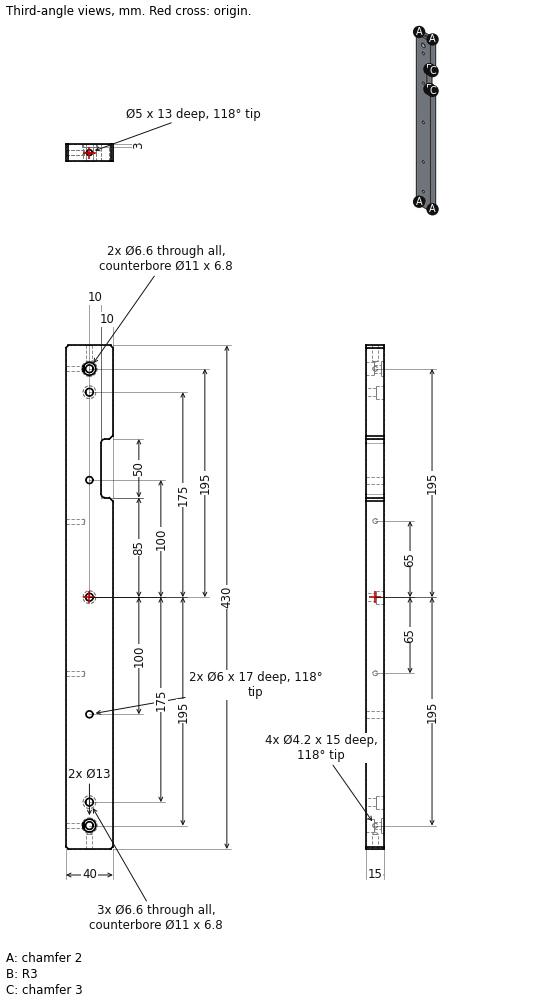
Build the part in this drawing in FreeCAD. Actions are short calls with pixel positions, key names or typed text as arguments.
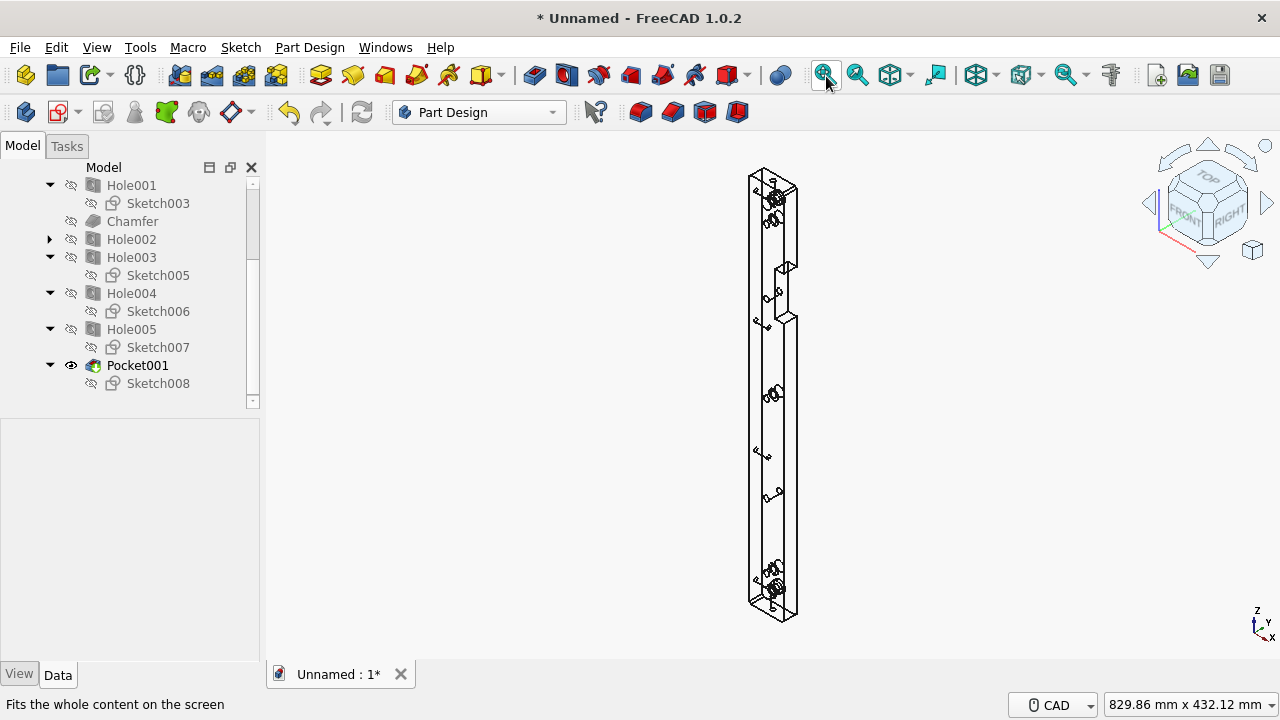
click(782, 314)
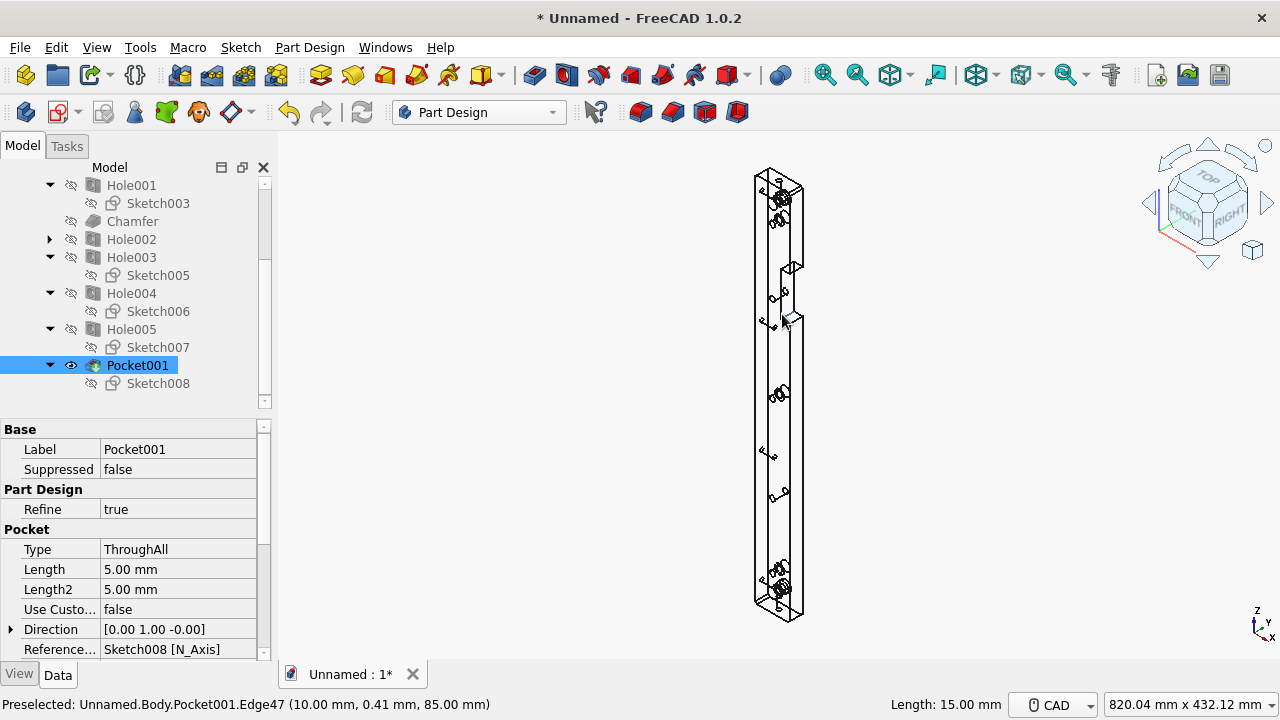
scroll(788, 264, up, 6)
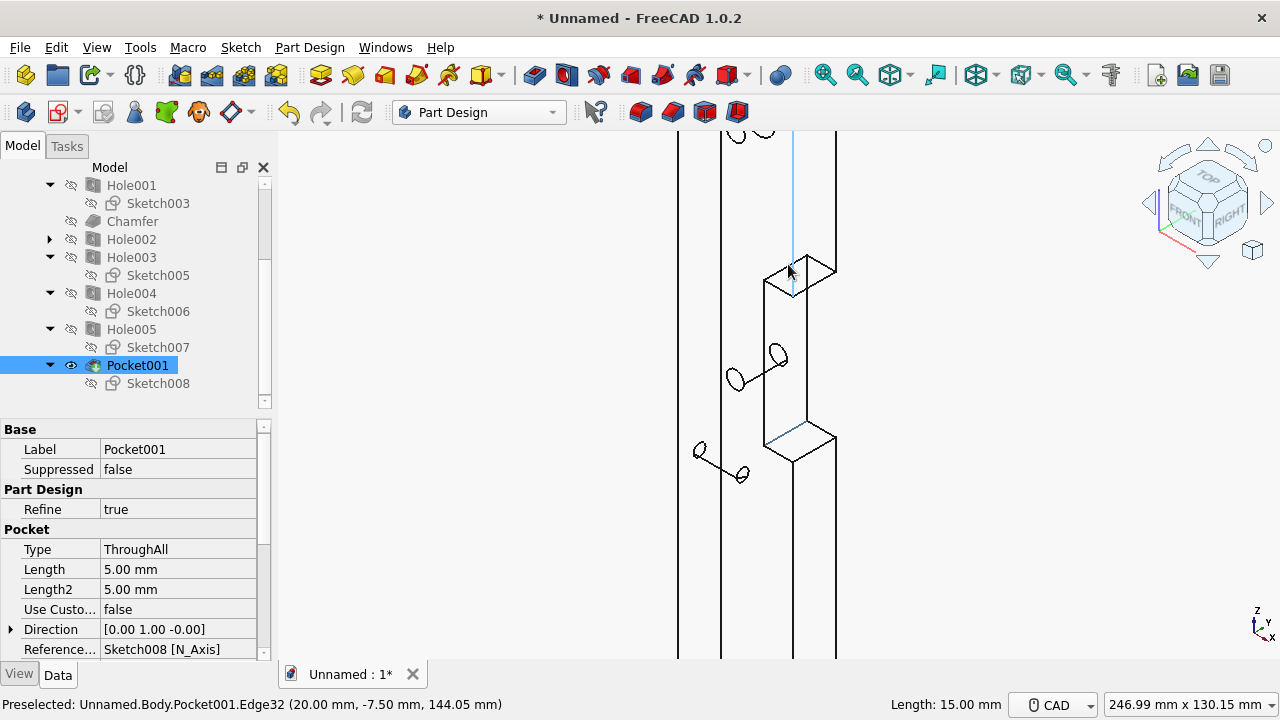
click(786, 267, ctrl)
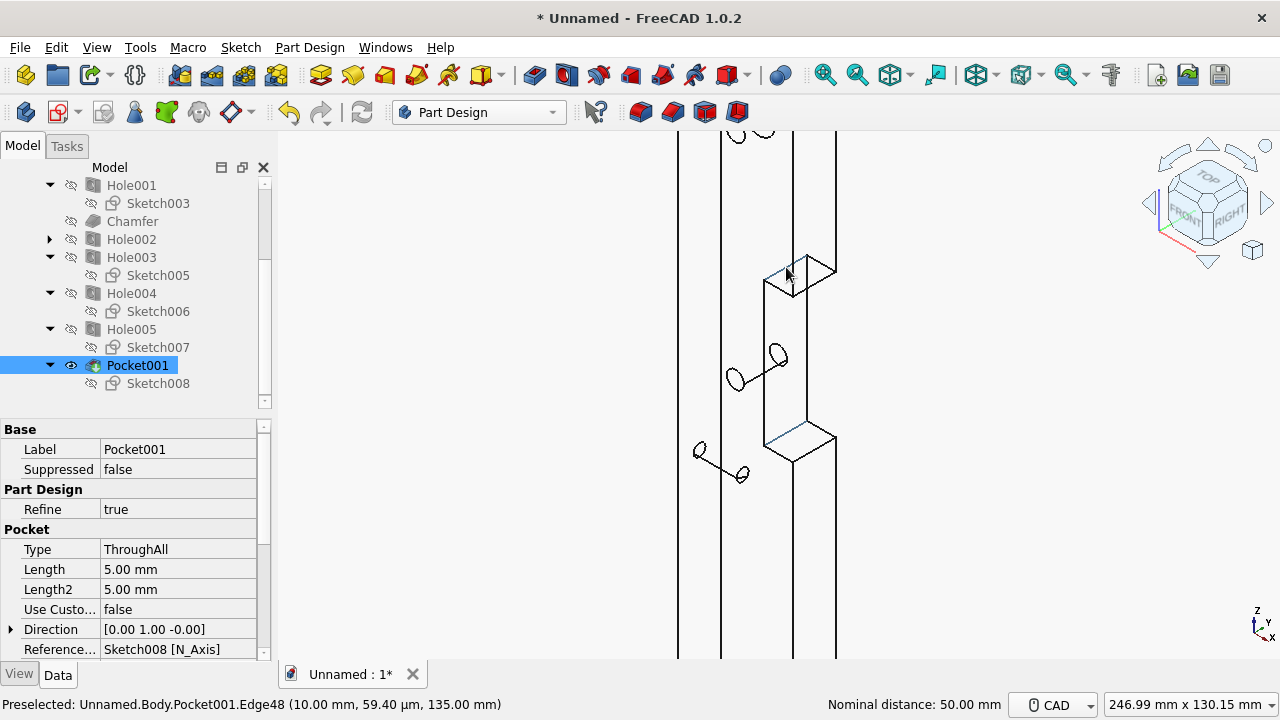
key(v)
key(1)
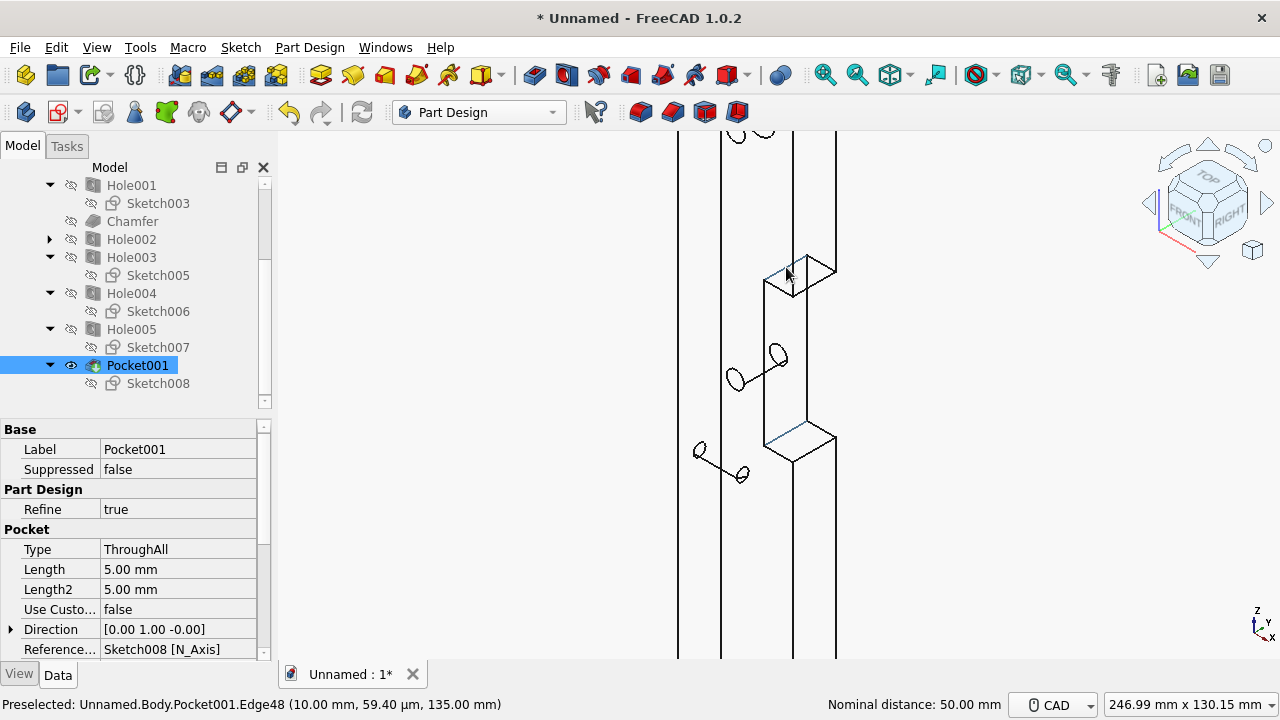
click(642, 112)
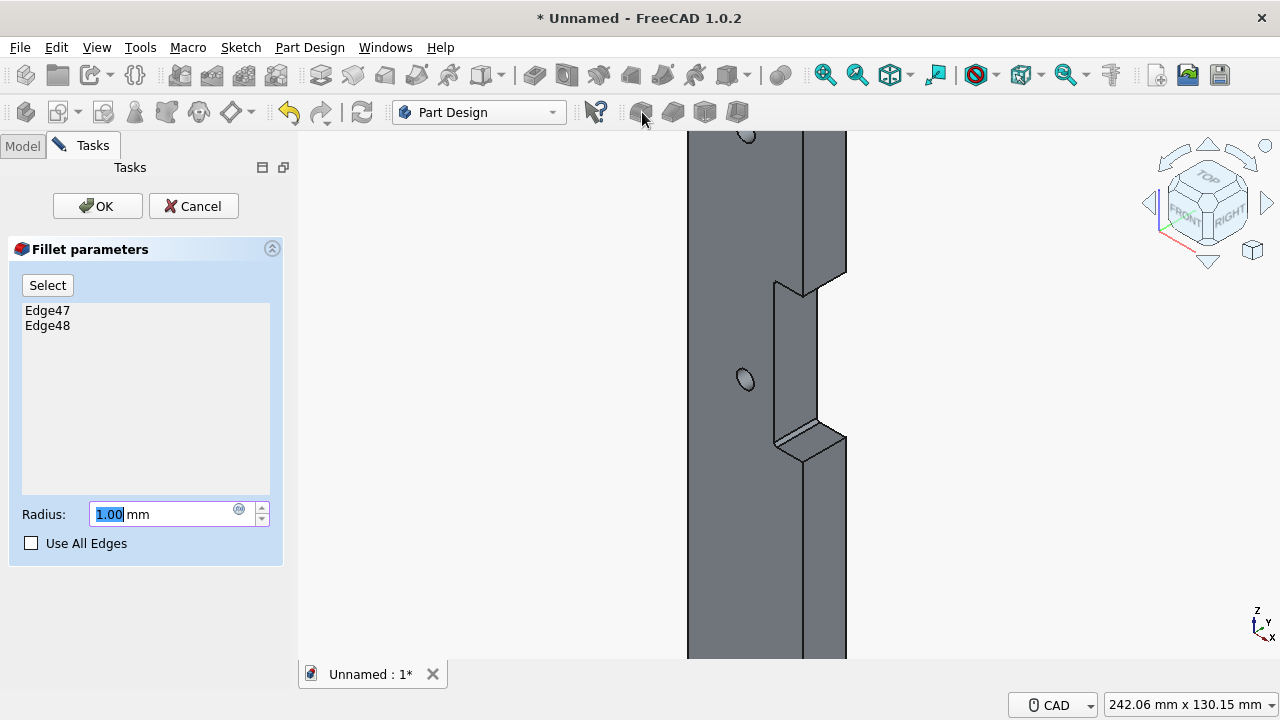
text(3)
key(Tab)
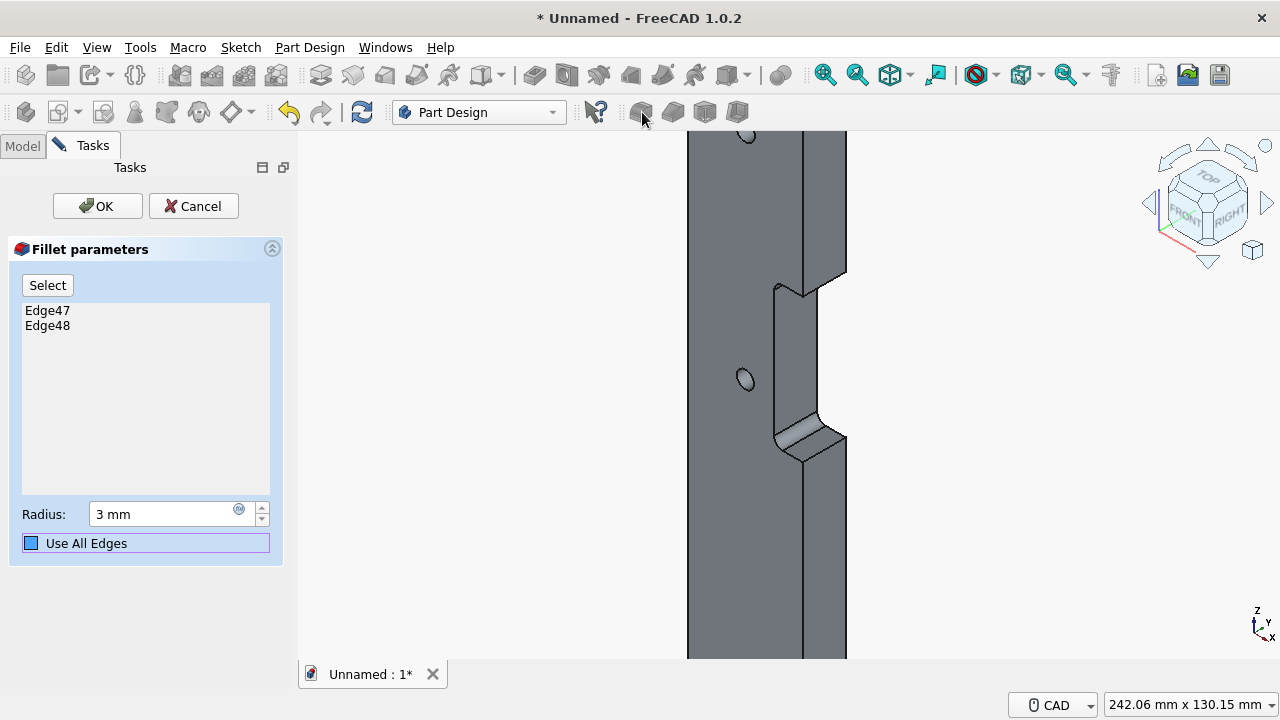
click(98, 206)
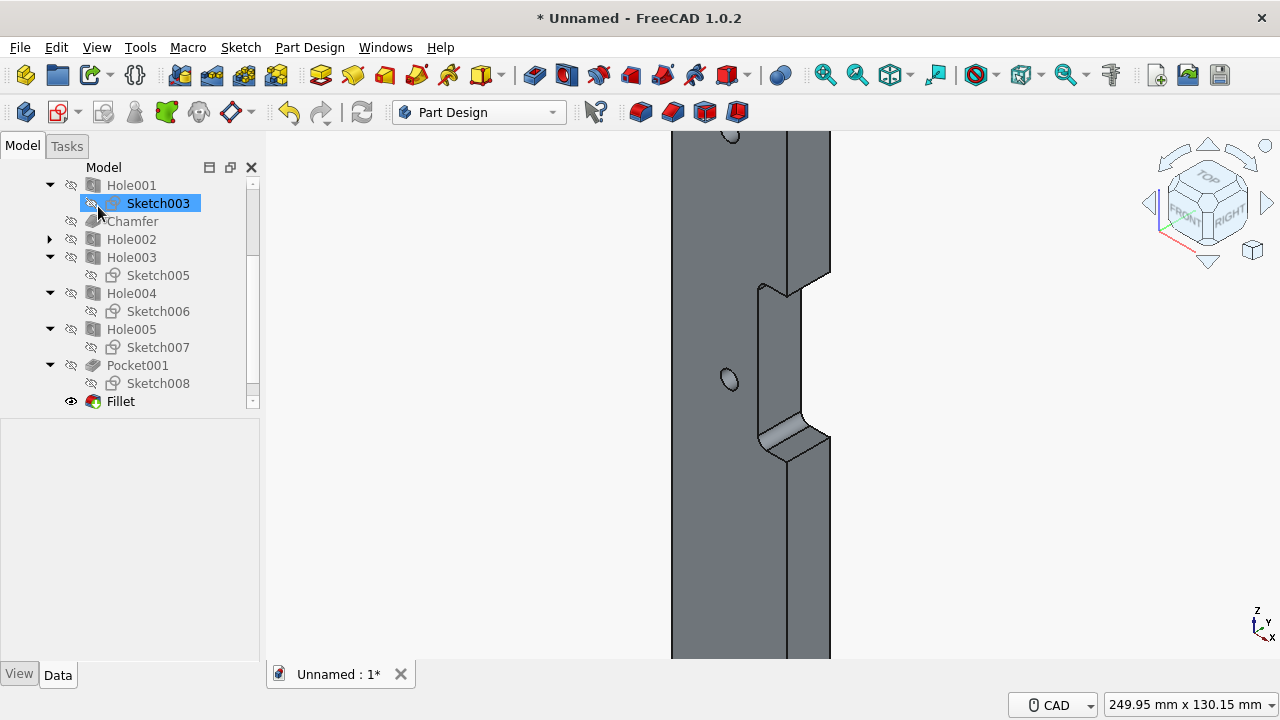
click(826, 76)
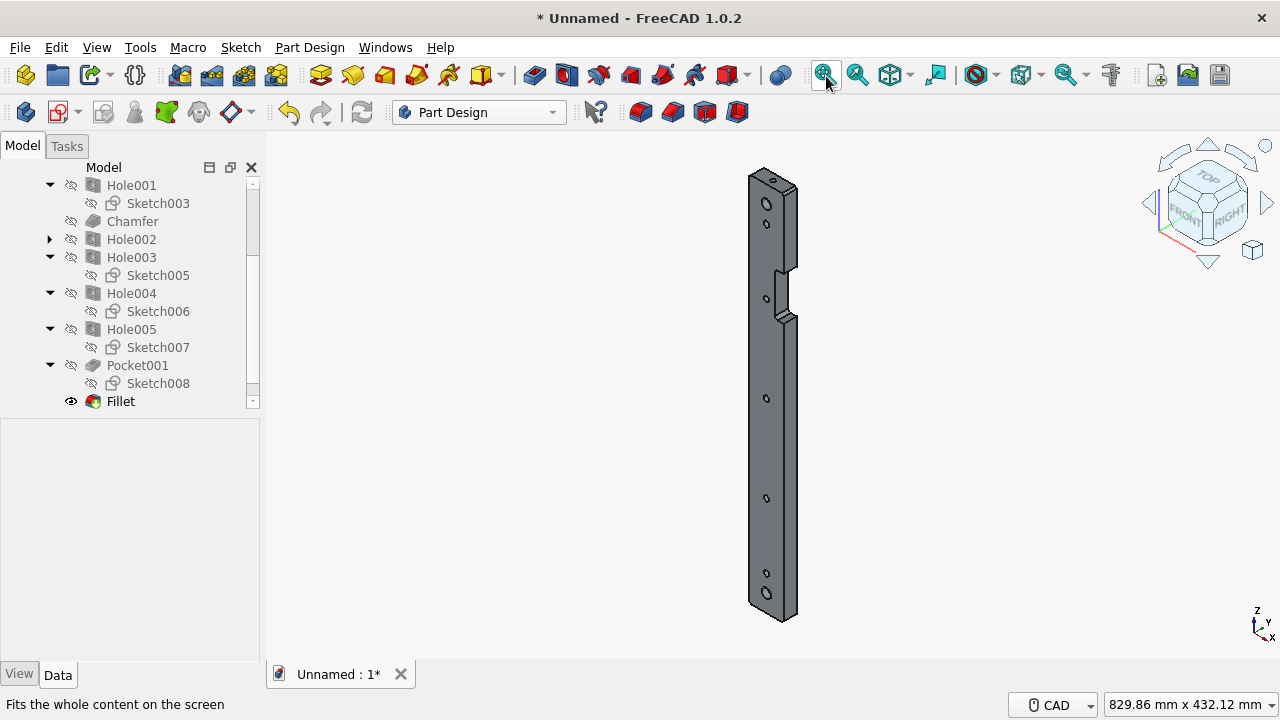
click(790, 319)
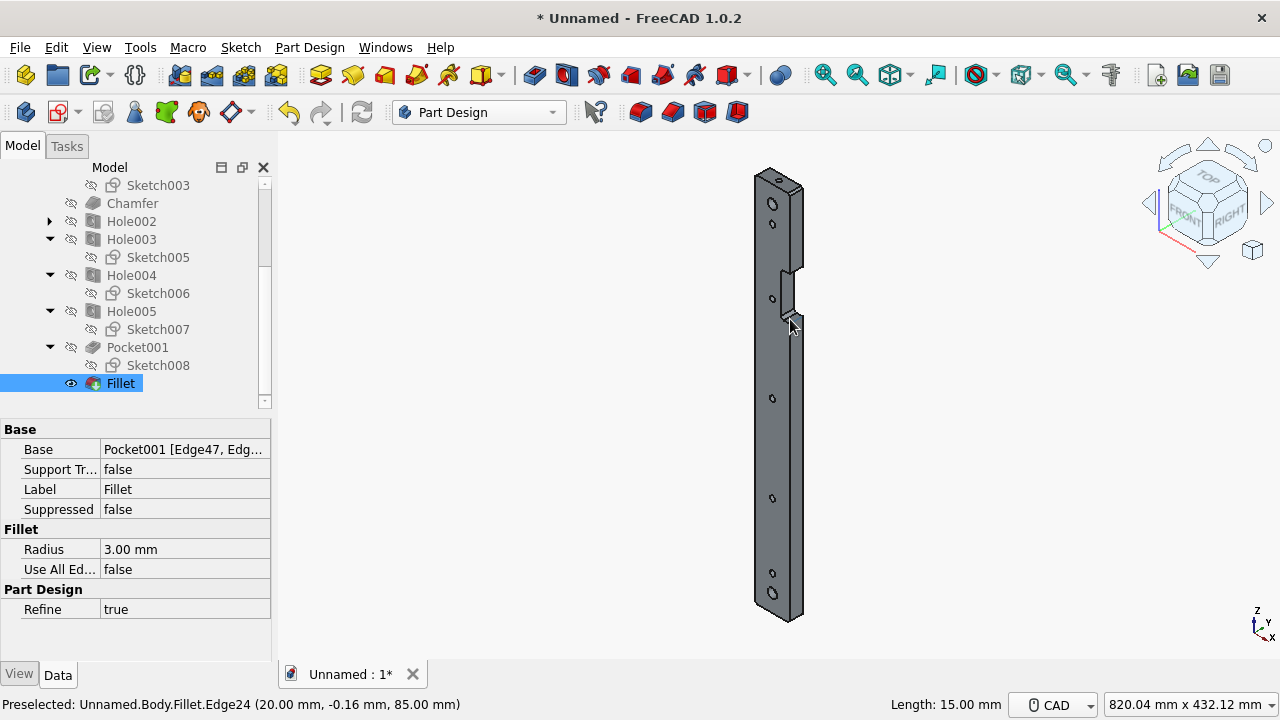
scroll(796, 269, up, 4)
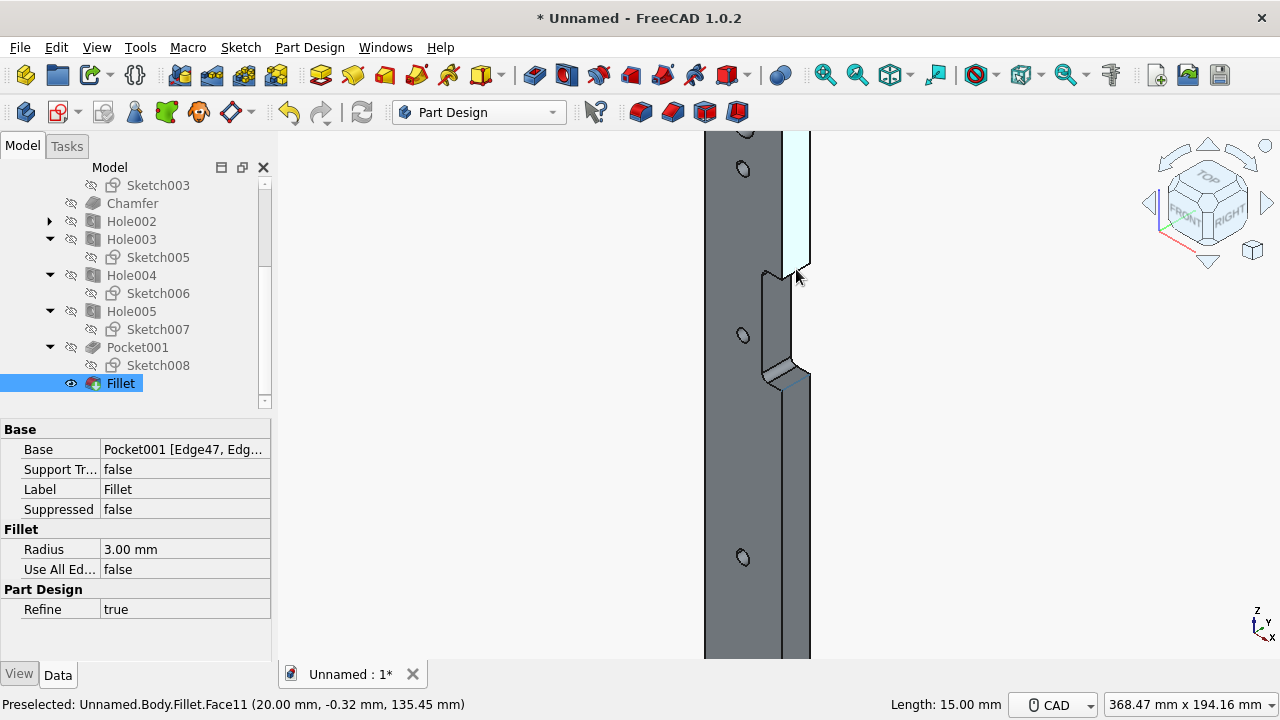
click(826, 76)